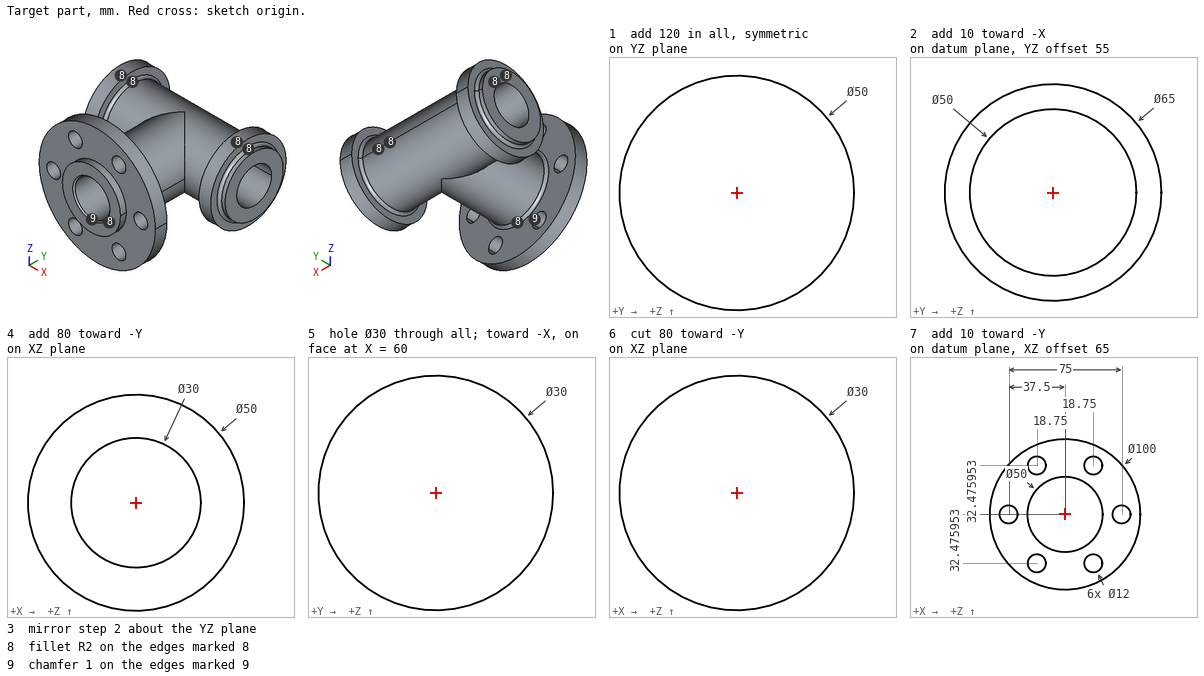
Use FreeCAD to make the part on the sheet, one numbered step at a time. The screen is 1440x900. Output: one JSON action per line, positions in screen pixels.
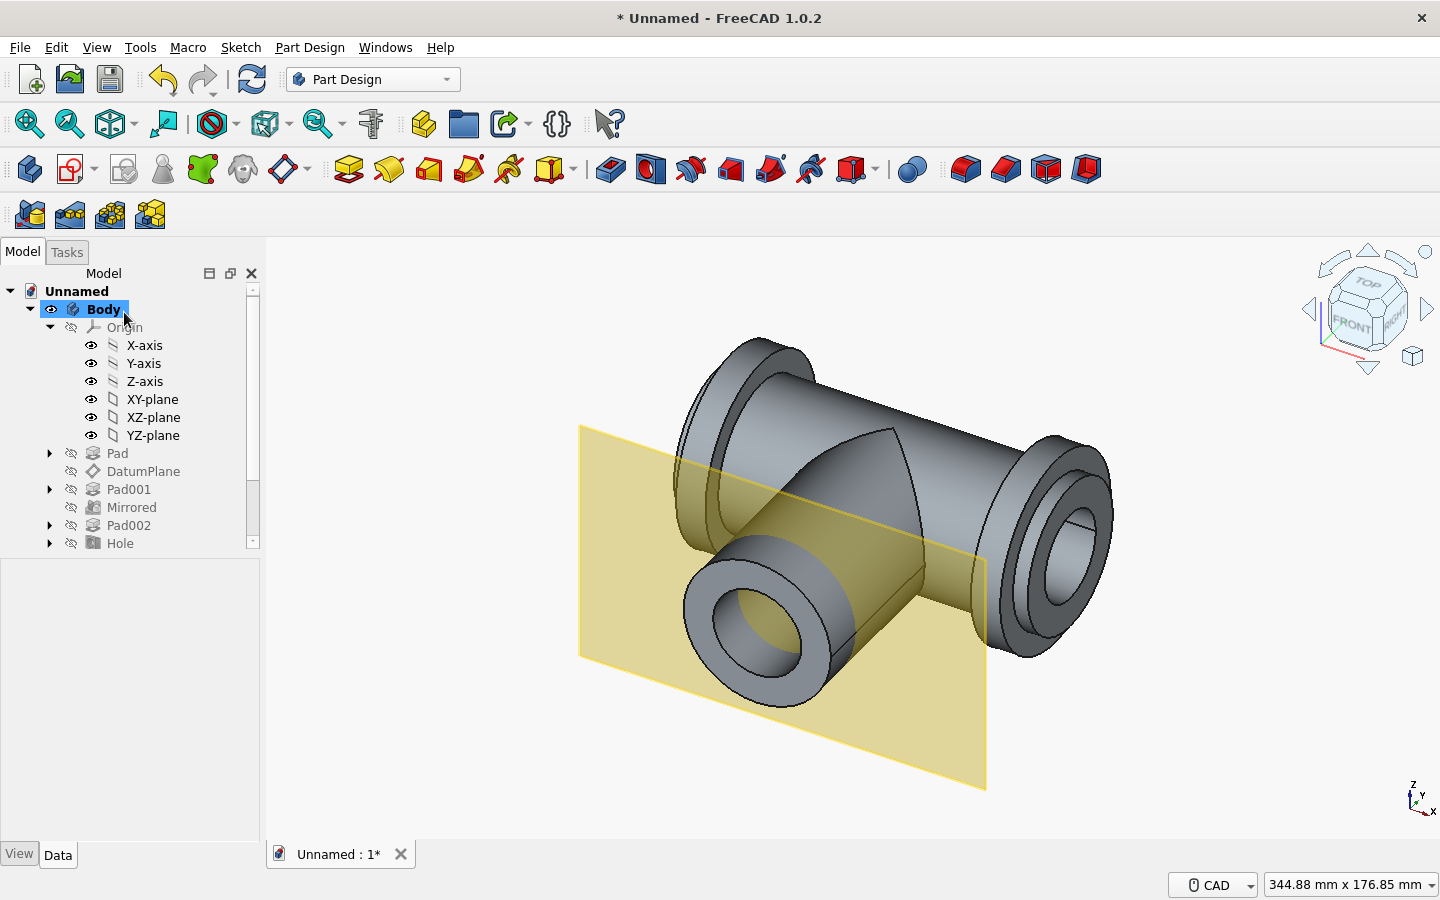
{"action": "scroll", "coordinate": [100, 413], "scroll_direction": "down", "scroll_amount": 3}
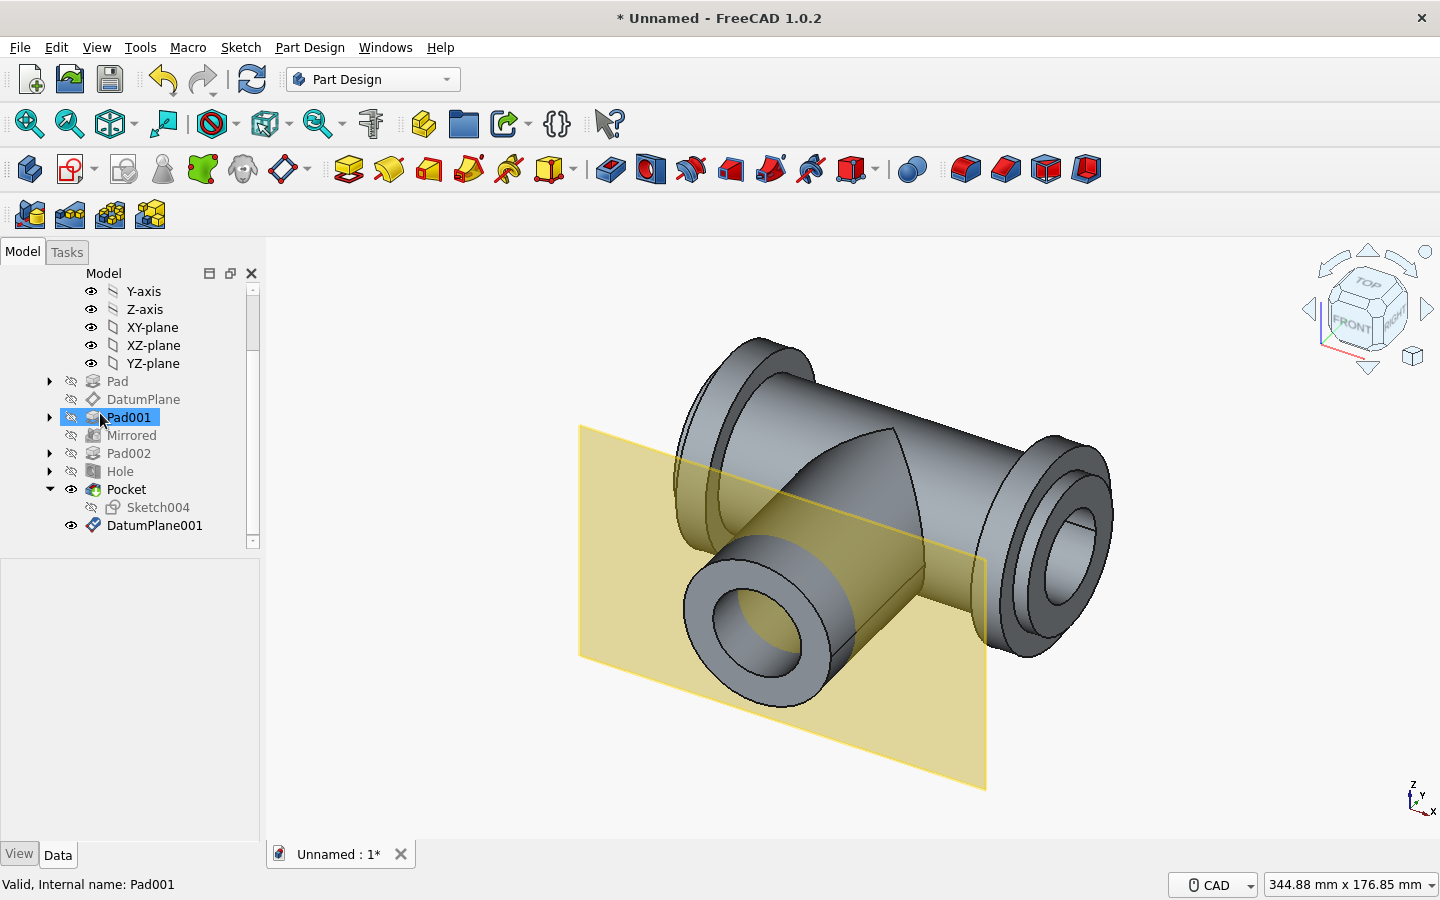
{"action": "left_click", "coordinate": [116, 525]}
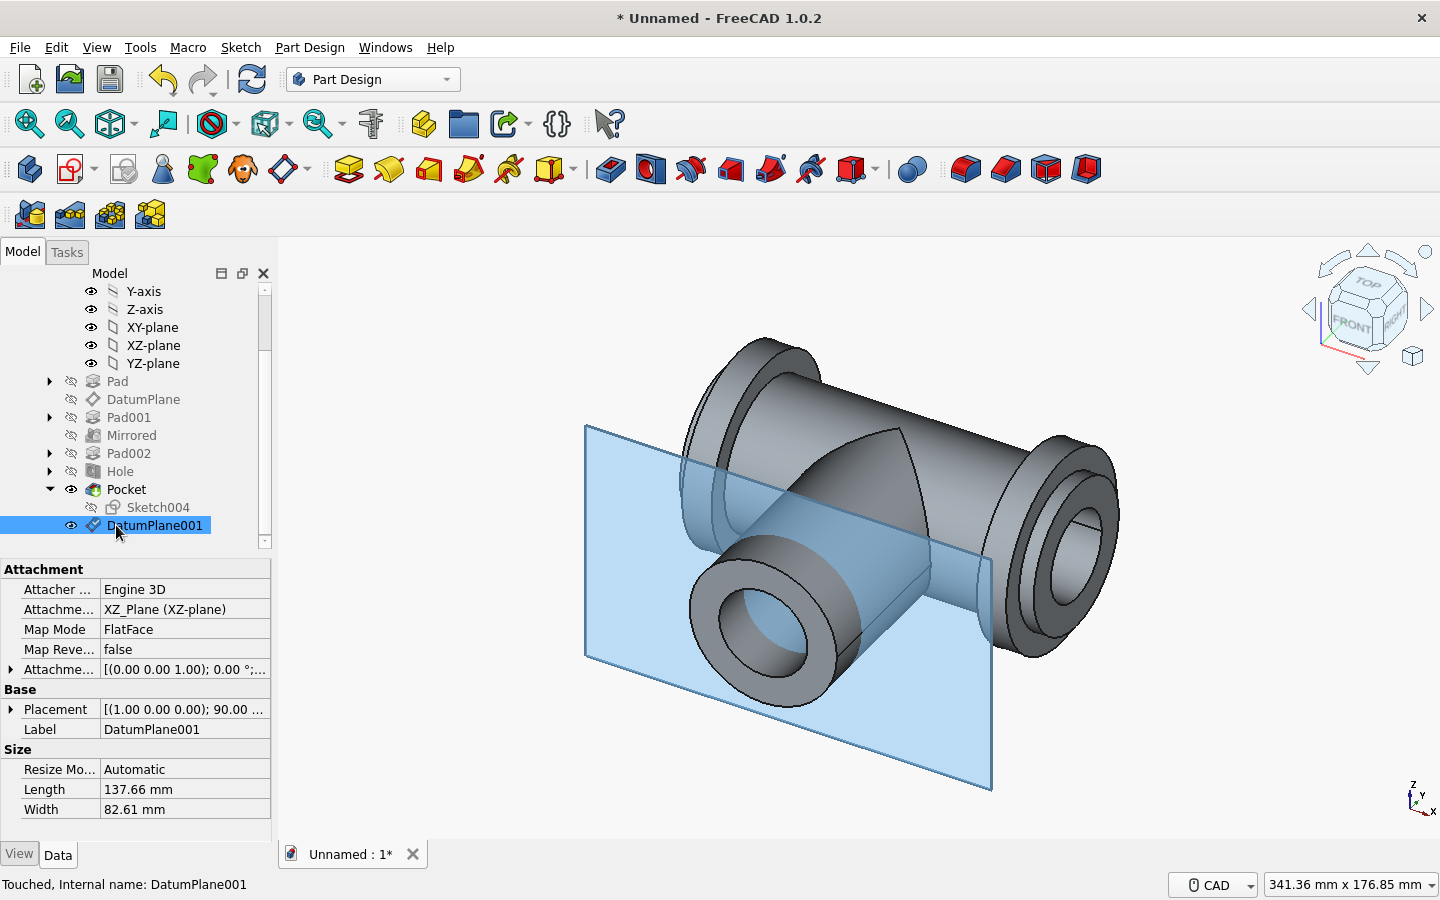
{"action": "left_click", "coordinate": [70, 170]}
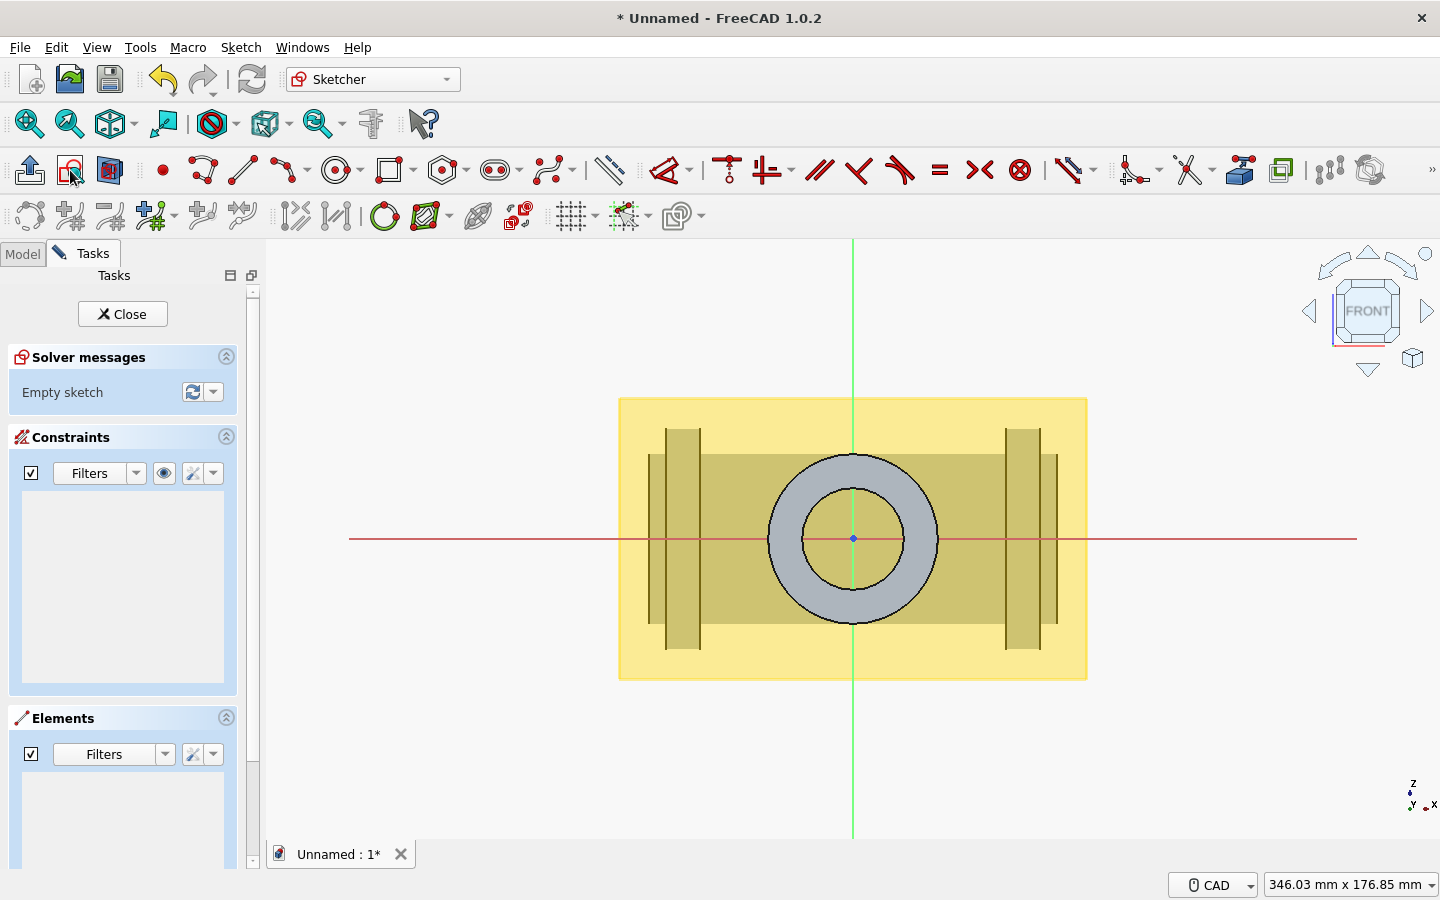
{"action": "left_click", "coordinate": [110, 170]}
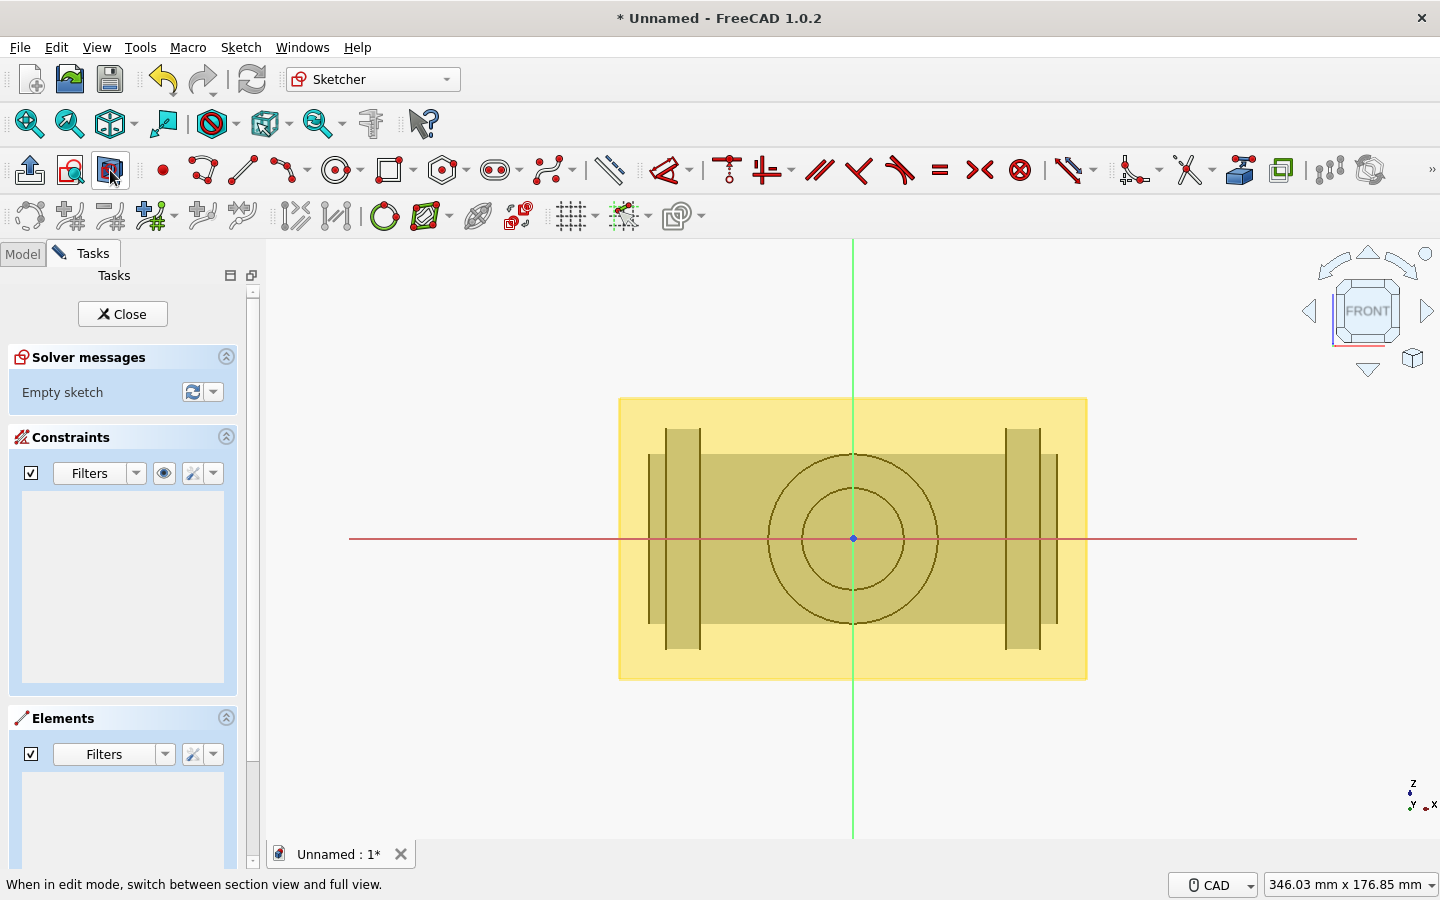
{"action": "key", "text": "g c"}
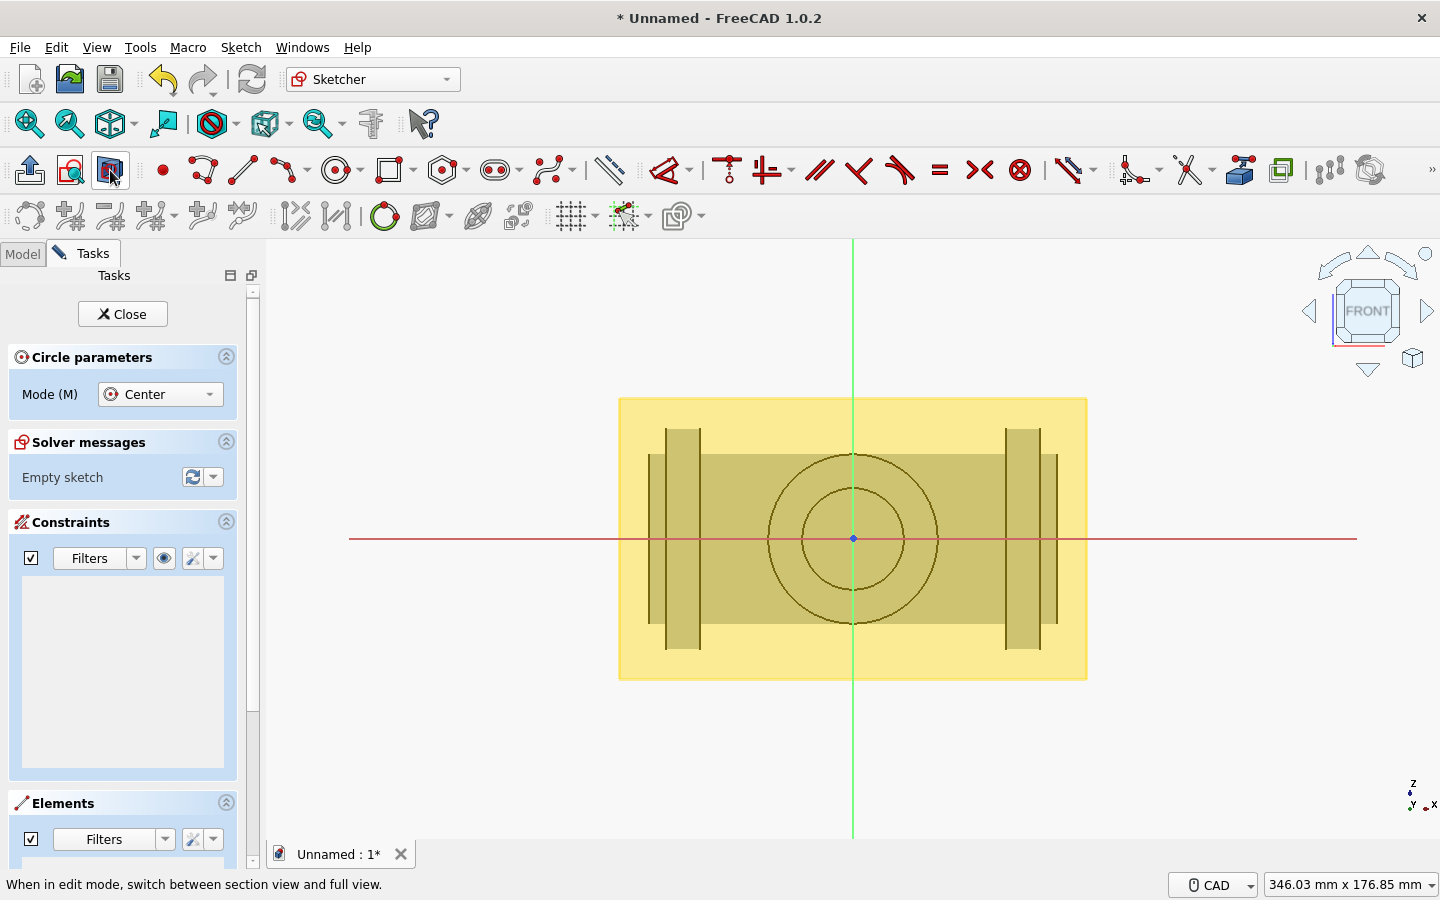
{"action": "left_click", "coordinate": [853, 539]}
{"action": "left_click", "coordinate": [973, 419]}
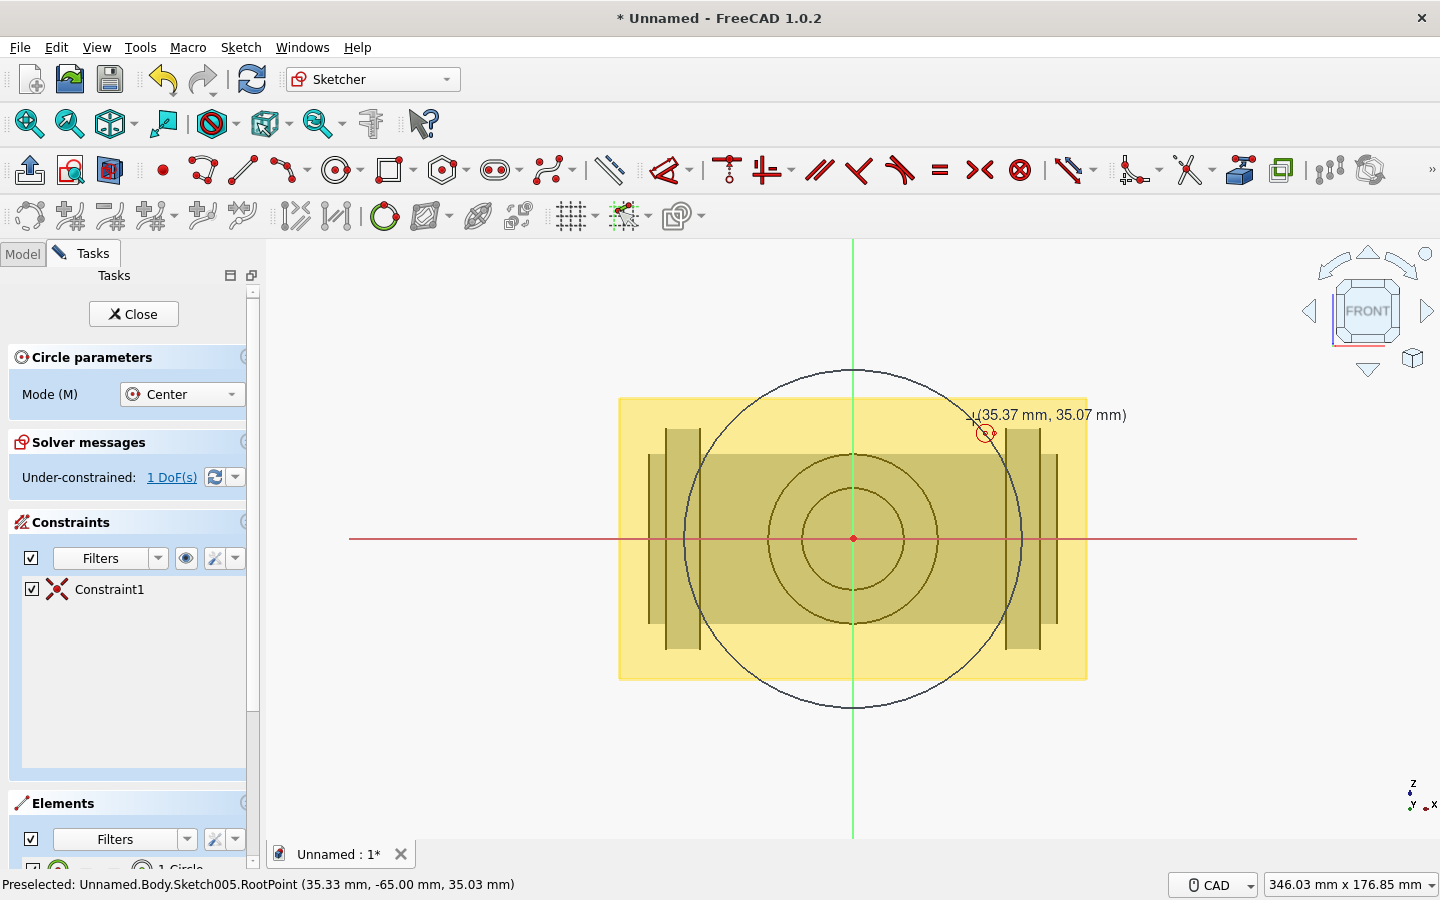
{"action": "left_click", "coordinate": [789, 429]}
{"action": "left_click", "coordinate": [804, 414]}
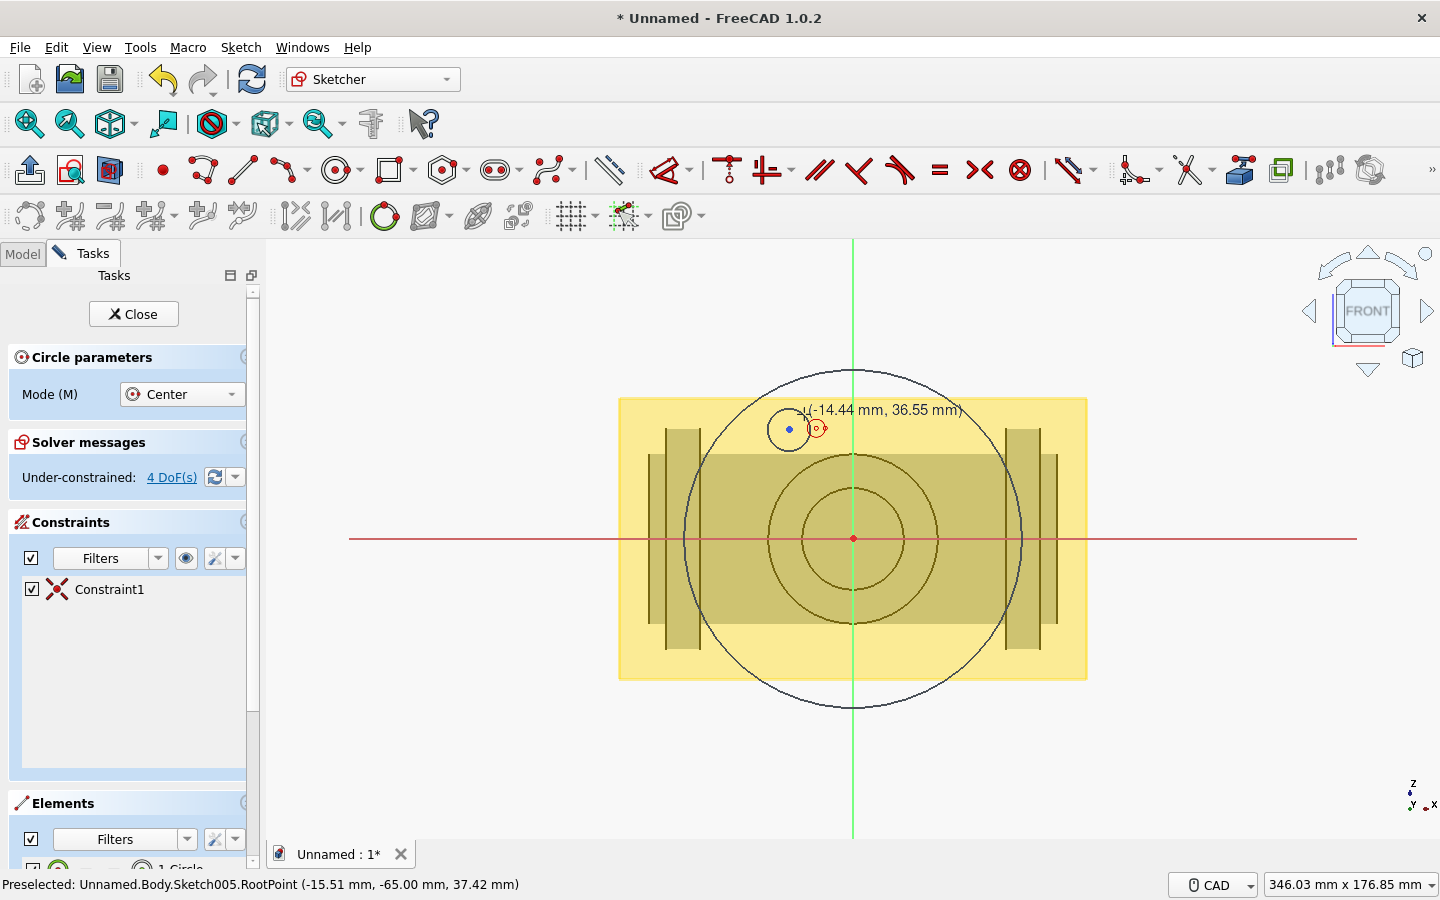
{"action": "left_click", "coordinate": [726, 539]}
{"action": "left_click", "coordinate": [740, 525]}